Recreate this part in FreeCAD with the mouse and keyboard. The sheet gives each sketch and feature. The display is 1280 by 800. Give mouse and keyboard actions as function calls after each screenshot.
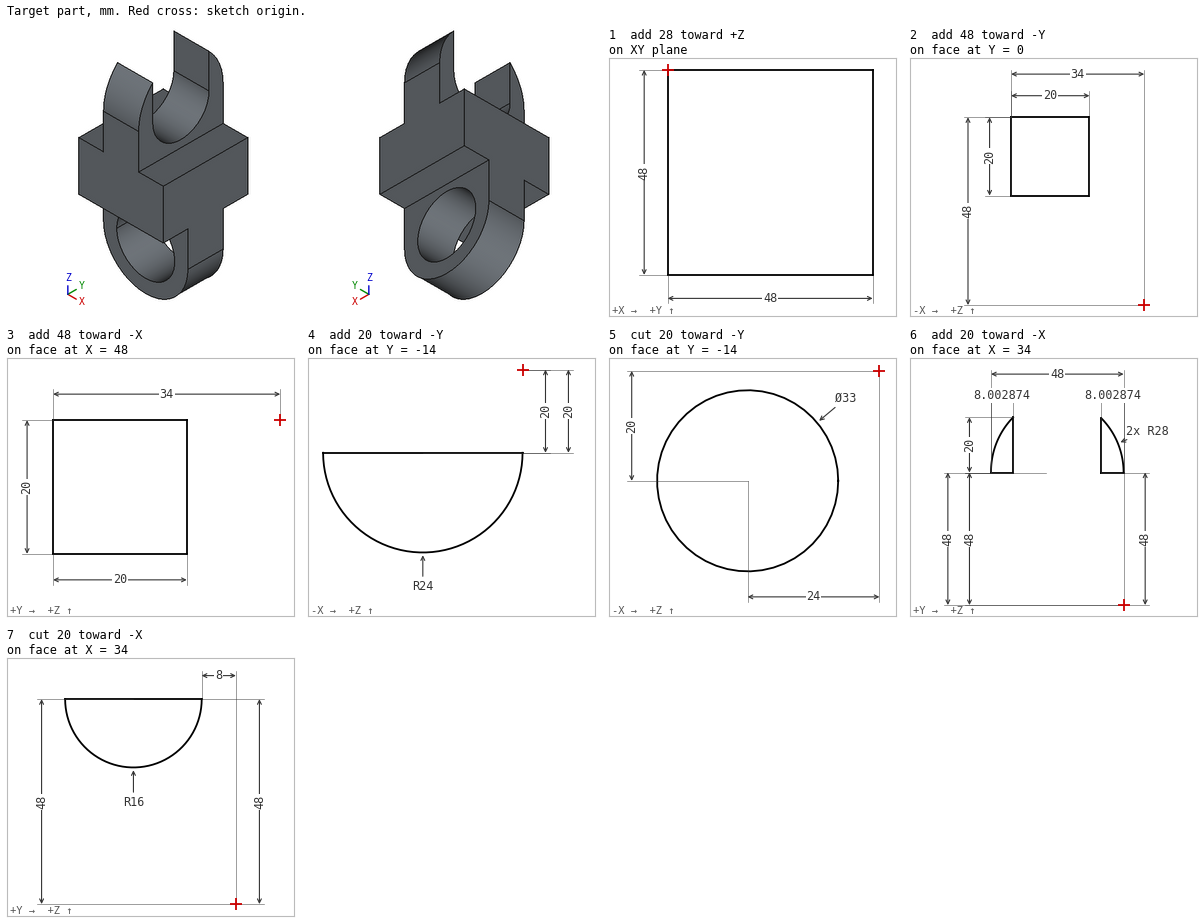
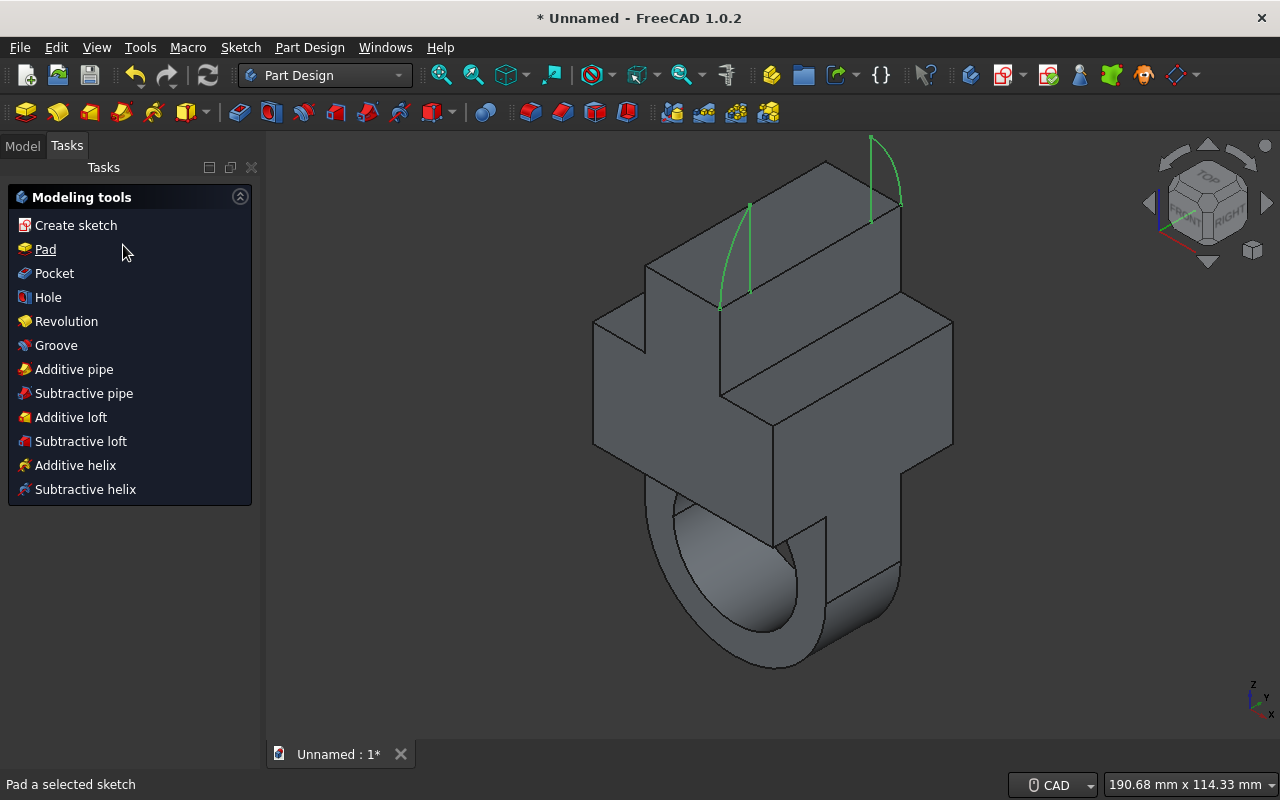
click(26, 112)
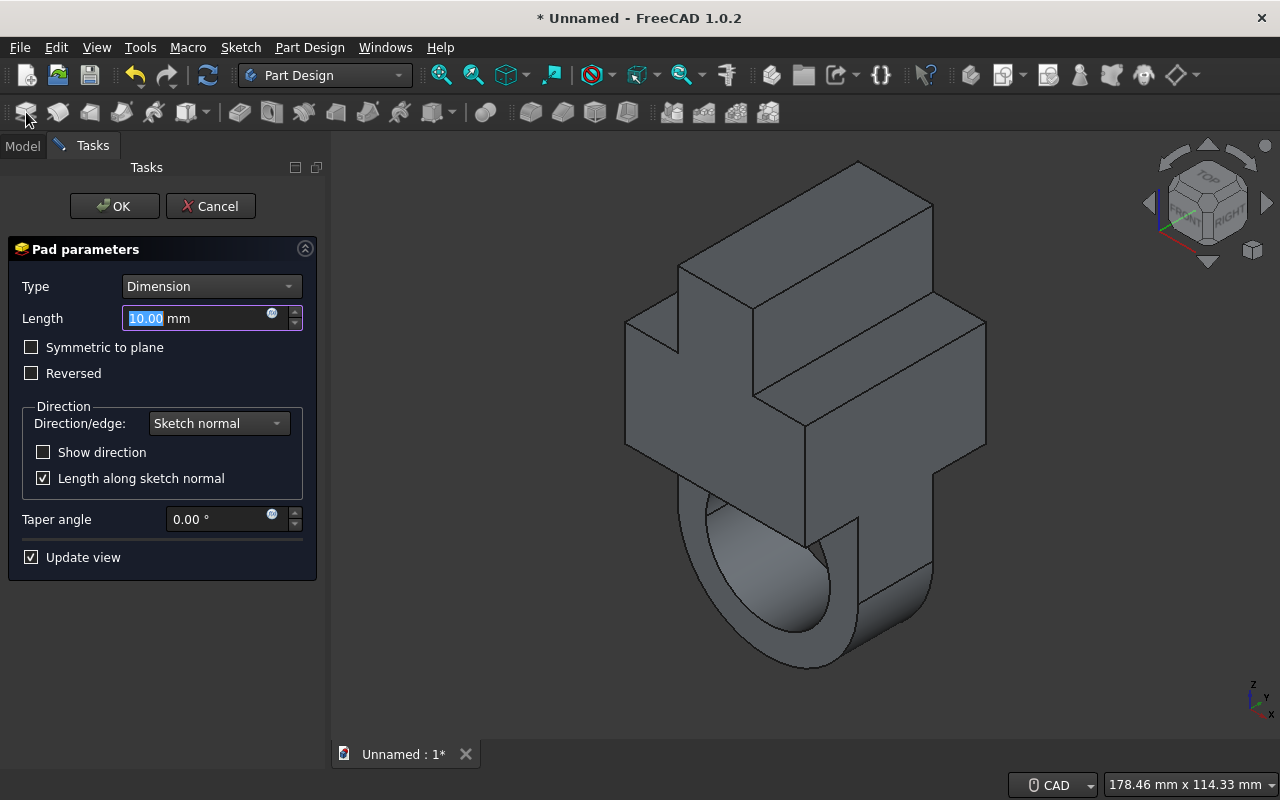
text(20)
key(Tab)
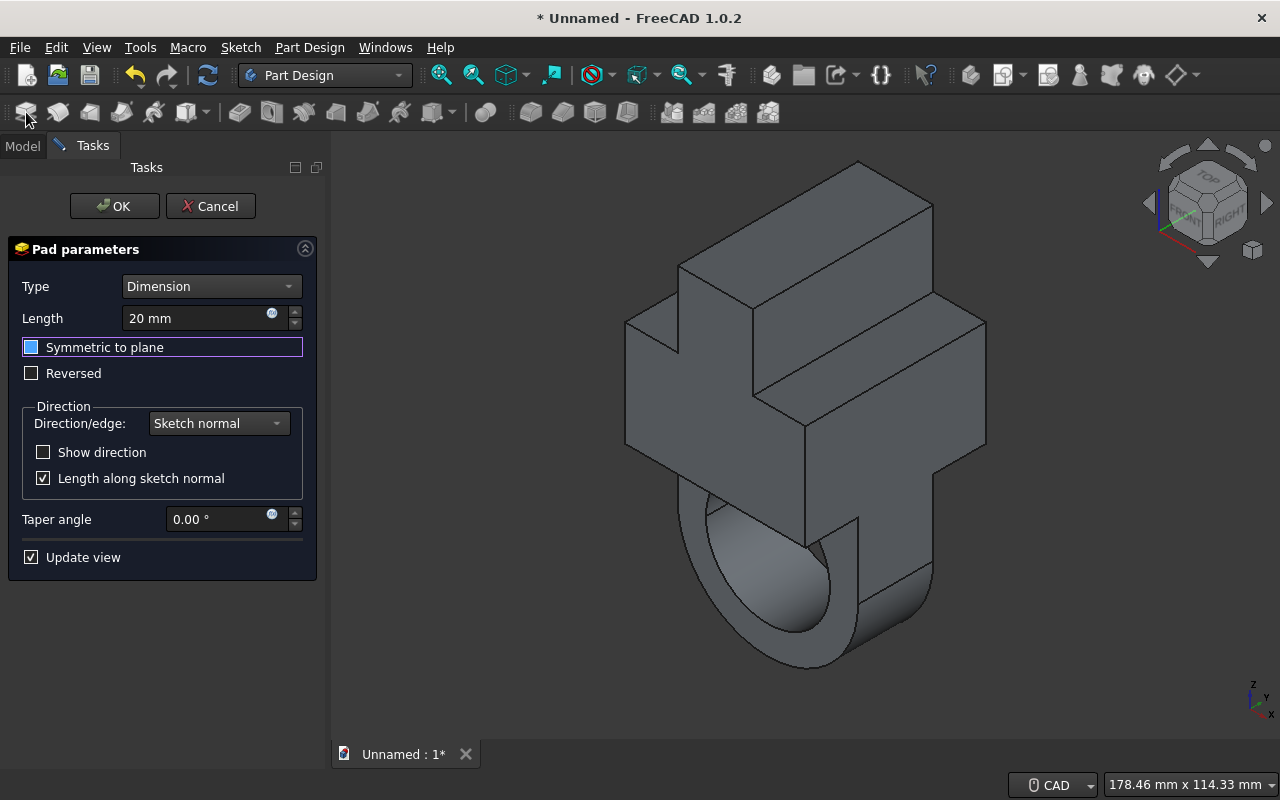
click(30, 373)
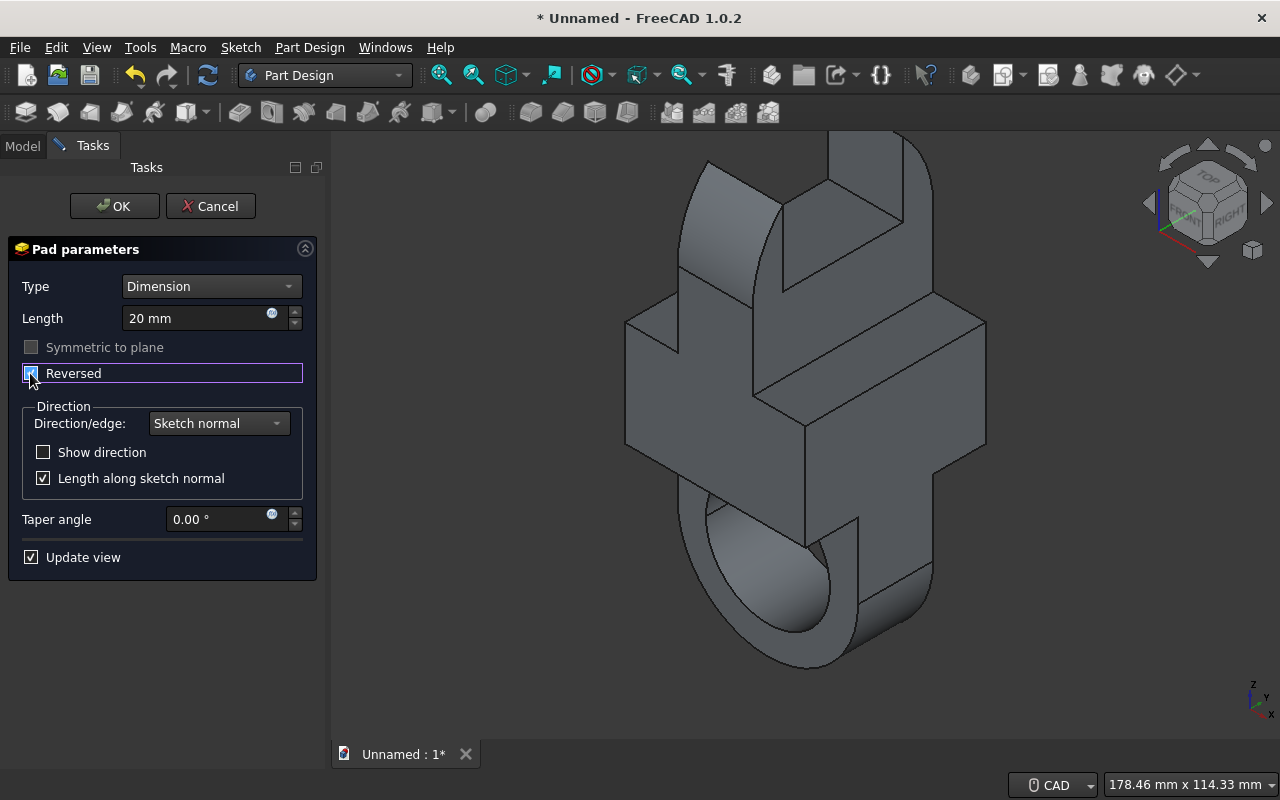
click(115, 206)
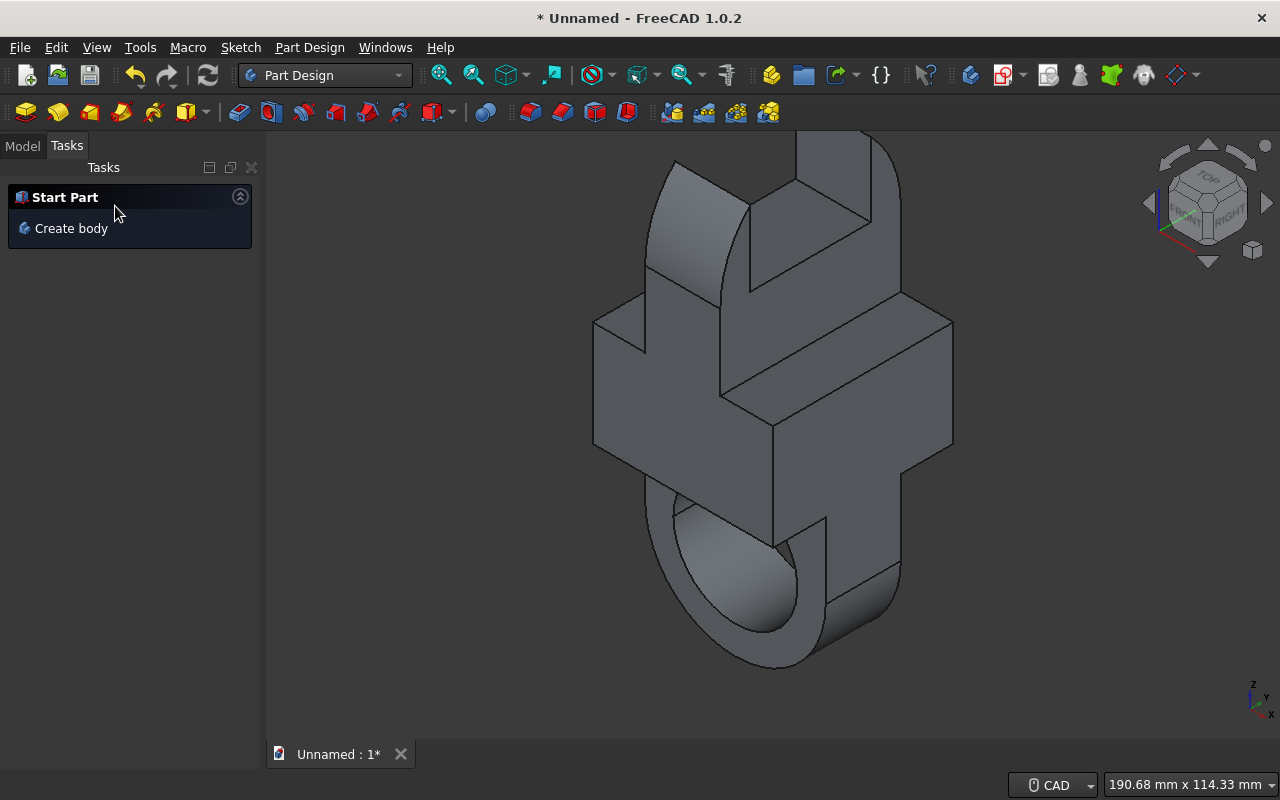
key(v)
key(f)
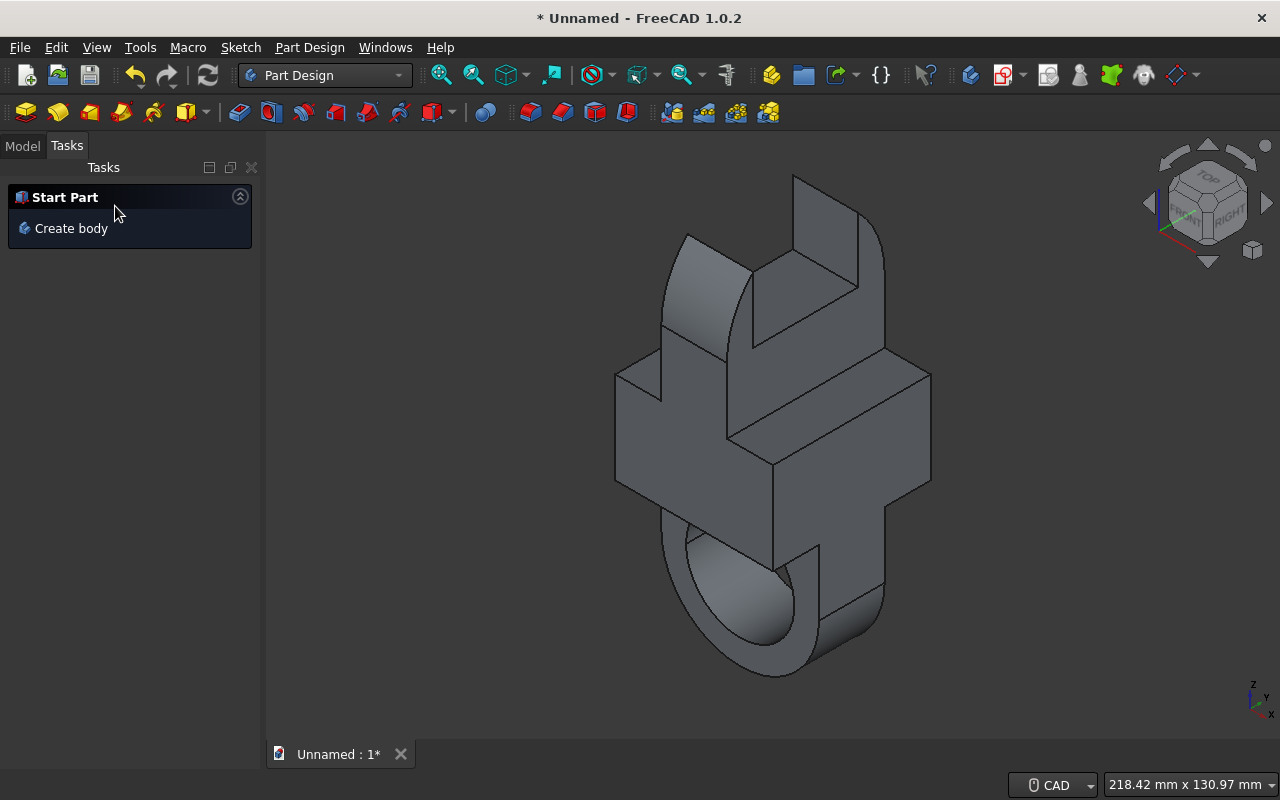
click(851, 334)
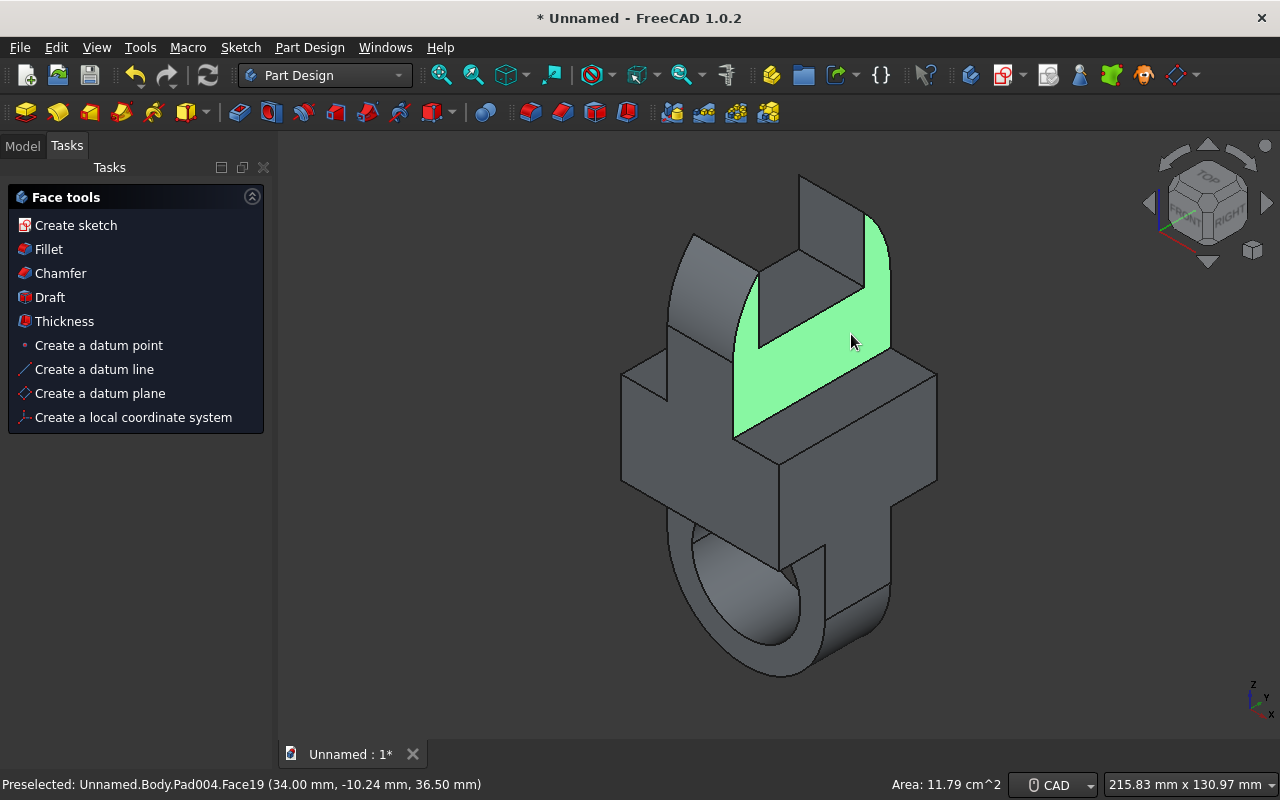
click(1004, 76)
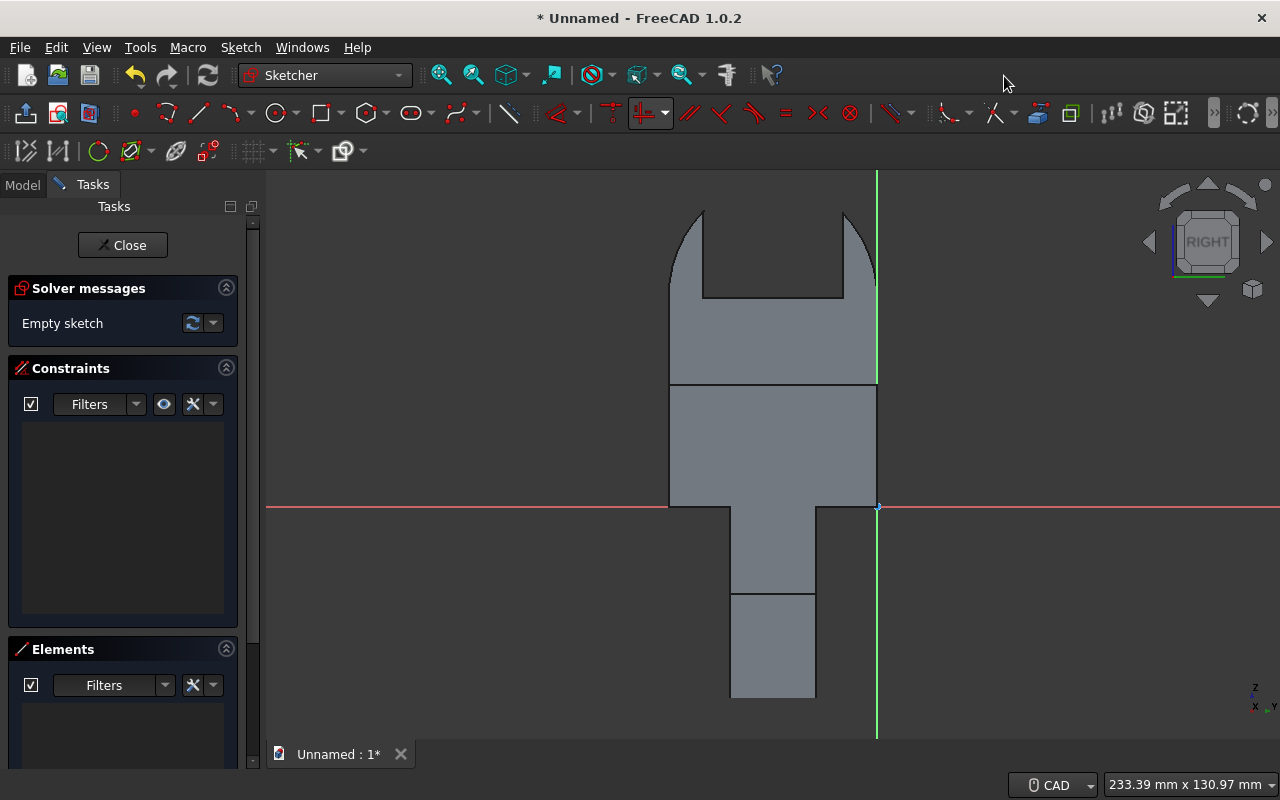
key(q)
key(s)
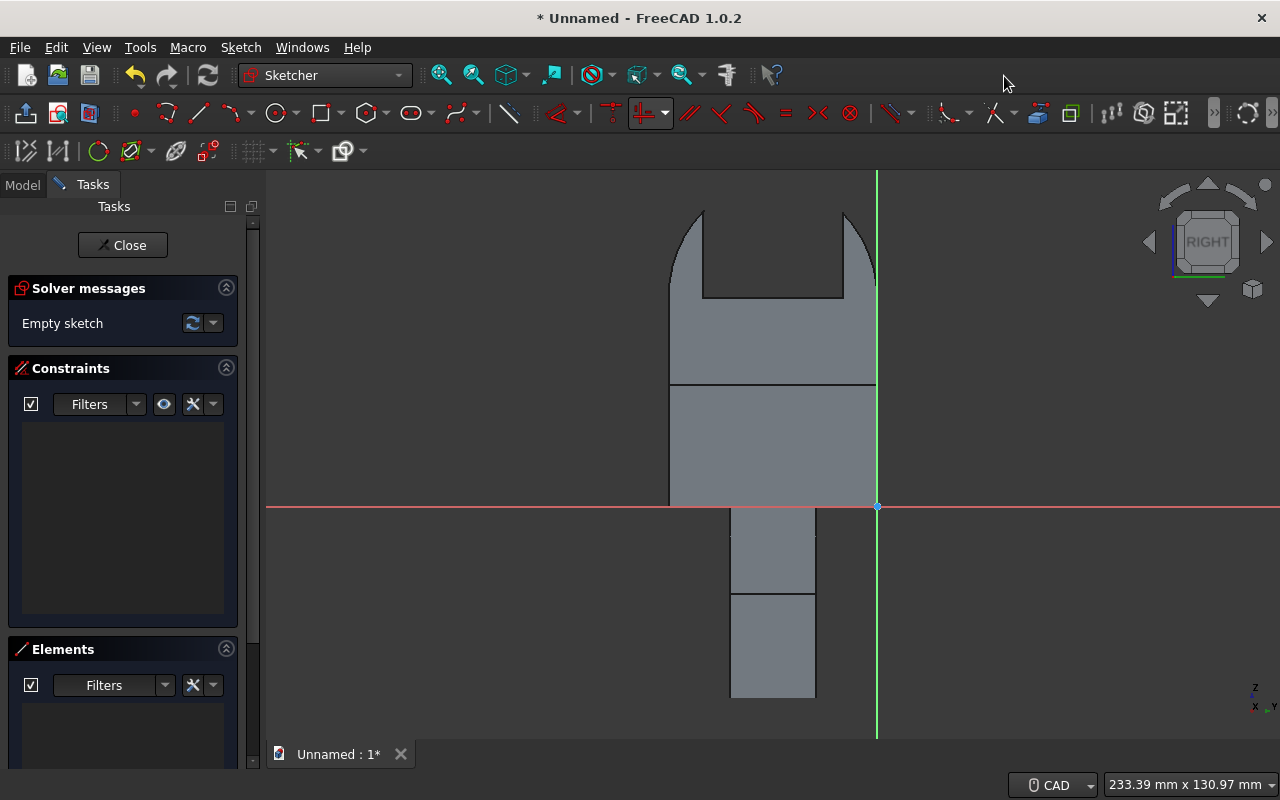
scroll(895, 339, up, 3)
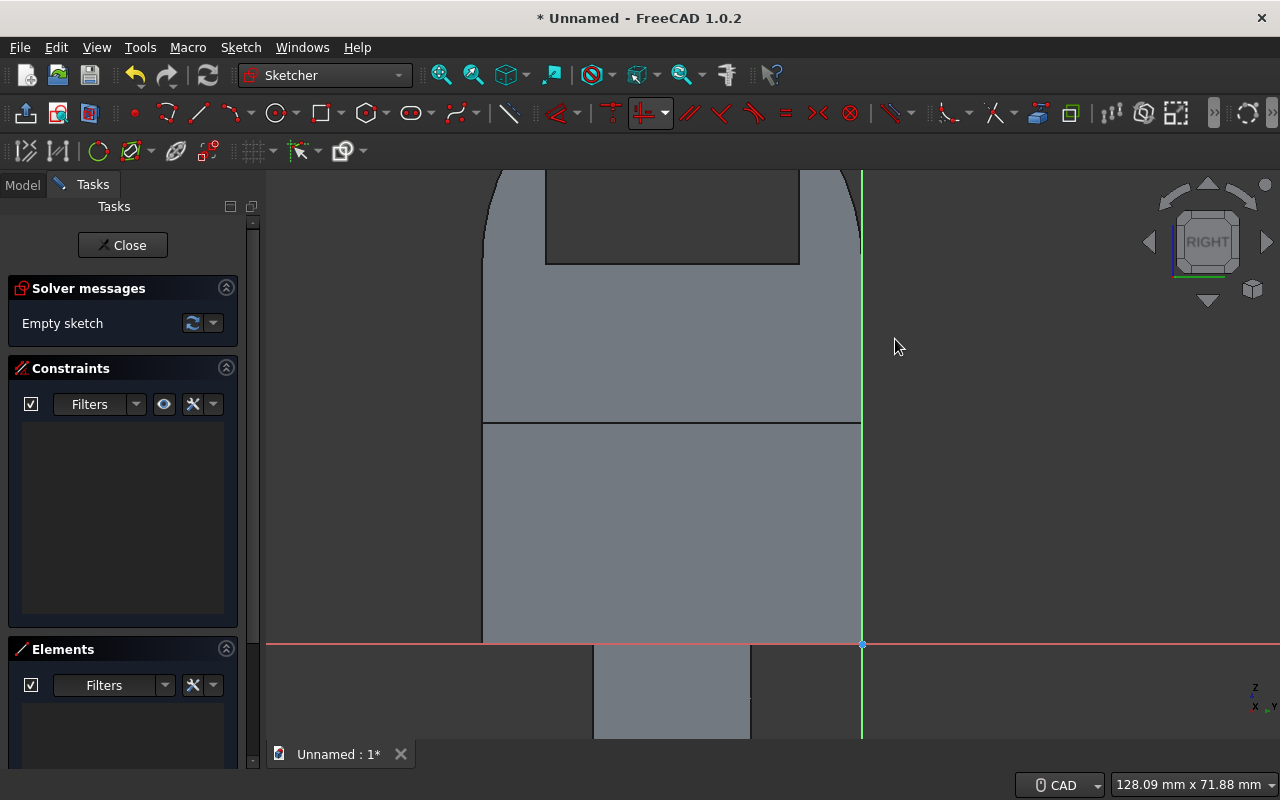
key(g)
key(l)